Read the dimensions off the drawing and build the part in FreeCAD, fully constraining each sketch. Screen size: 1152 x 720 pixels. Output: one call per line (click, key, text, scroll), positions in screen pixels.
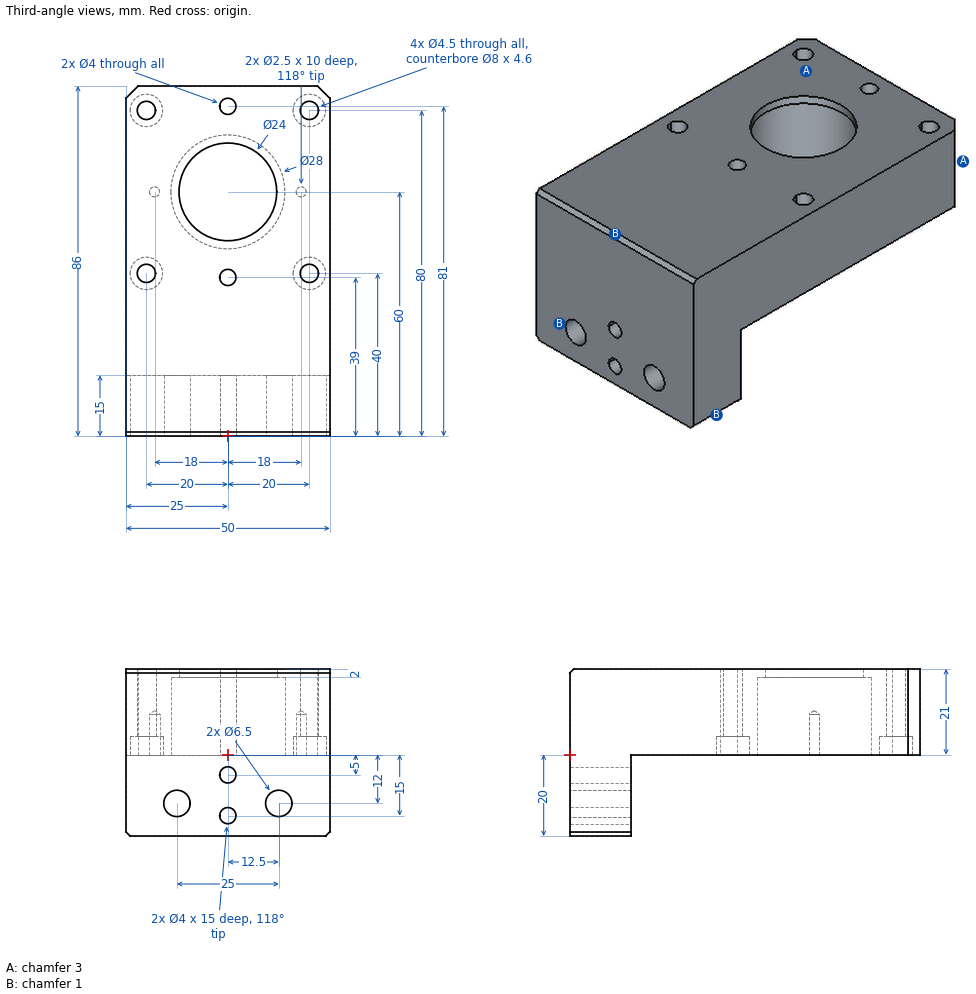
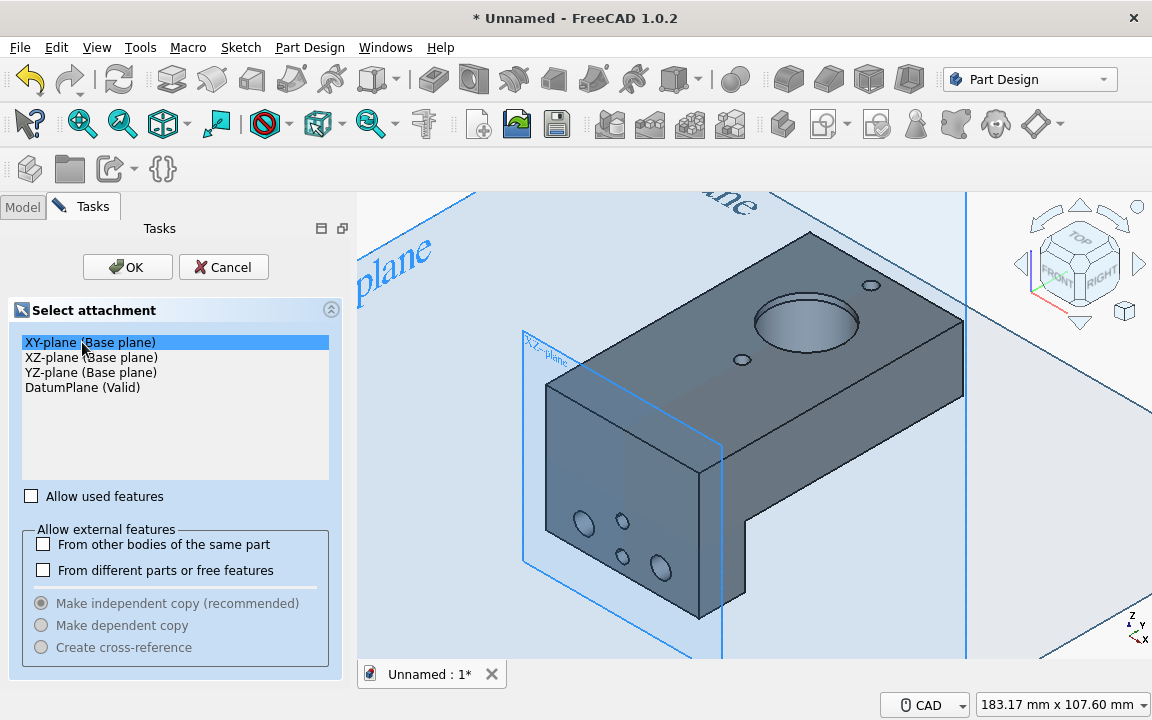
click(128, 267)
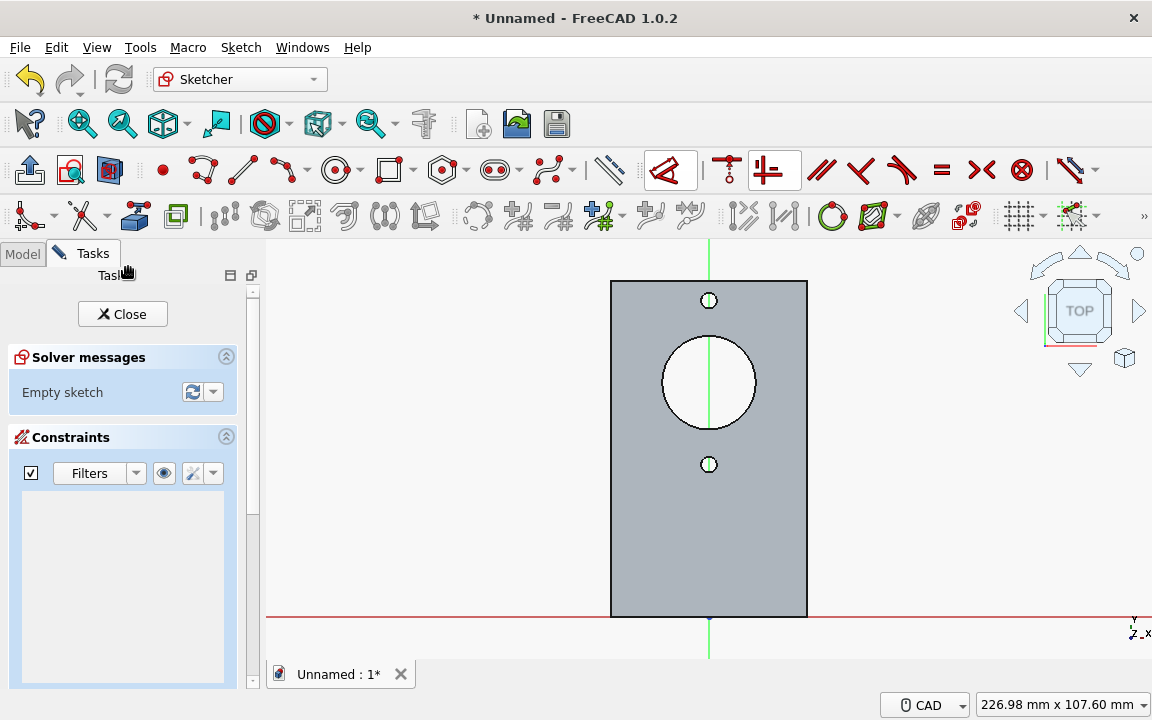
click(110, 170)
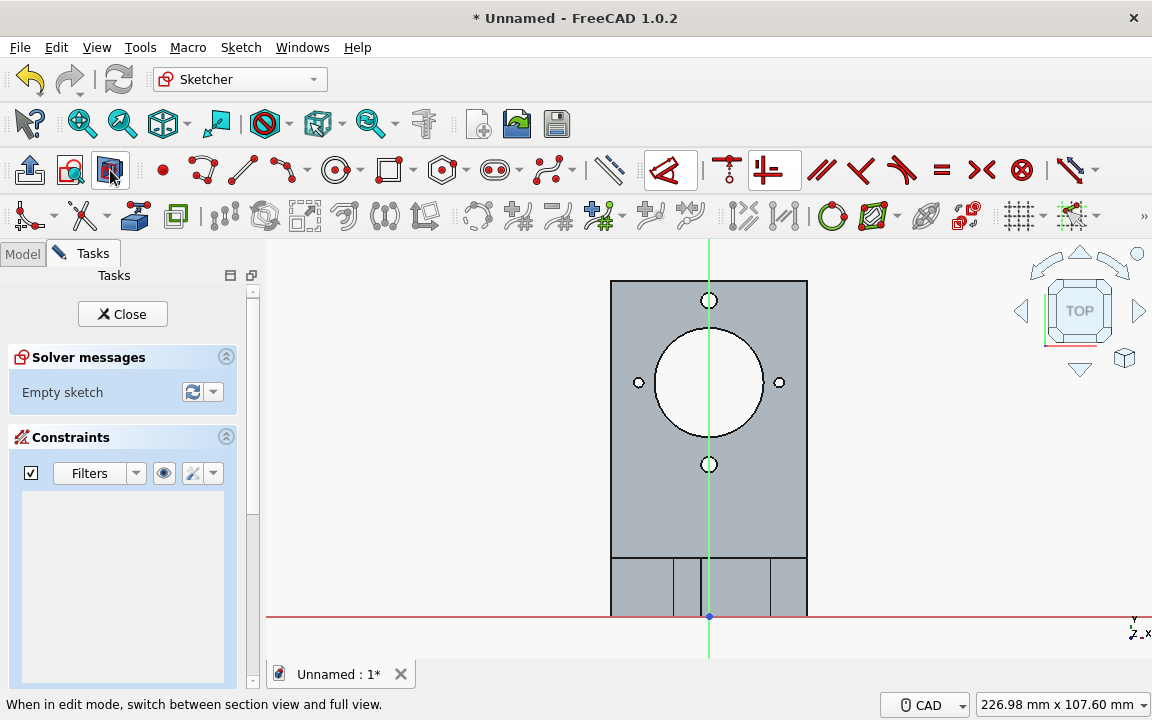
scroll(331, 416, down, 1)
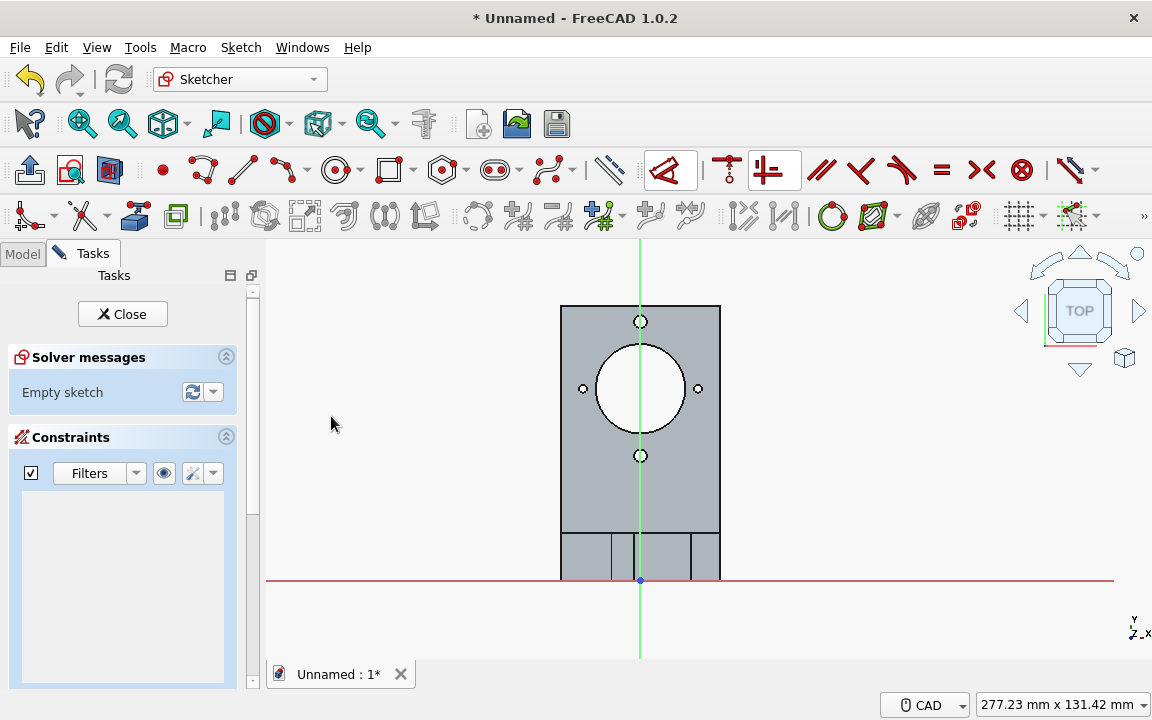
click(336, 170)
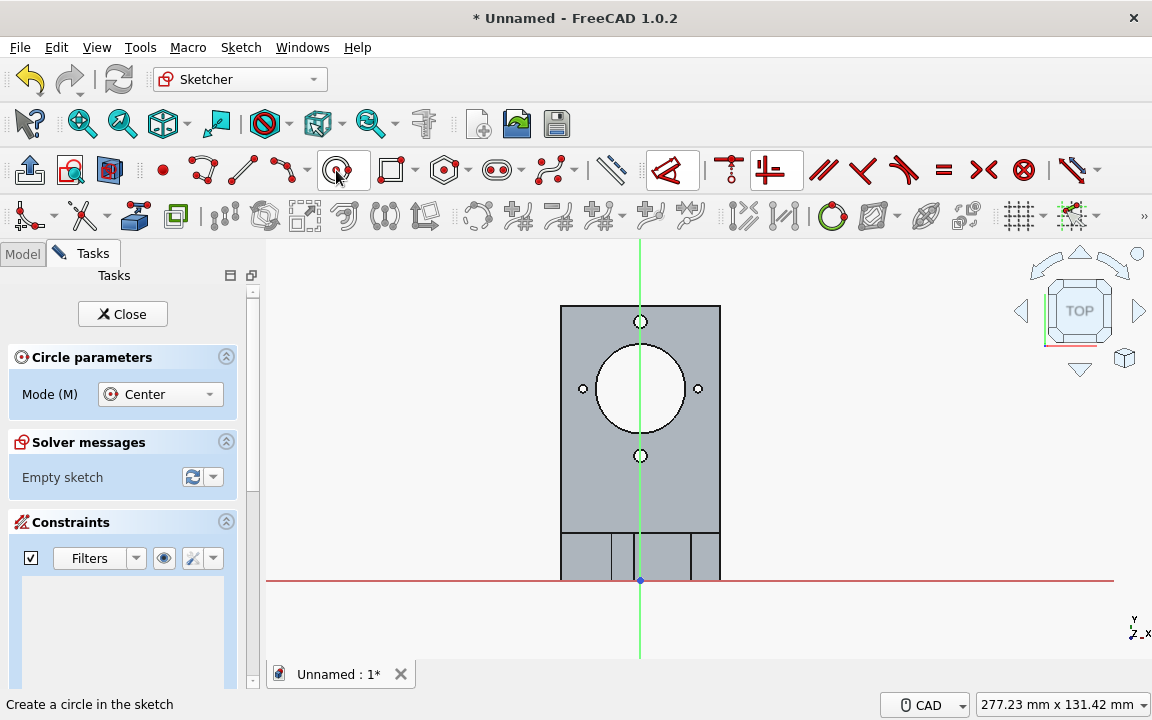
scroll(704, 325, up, 6)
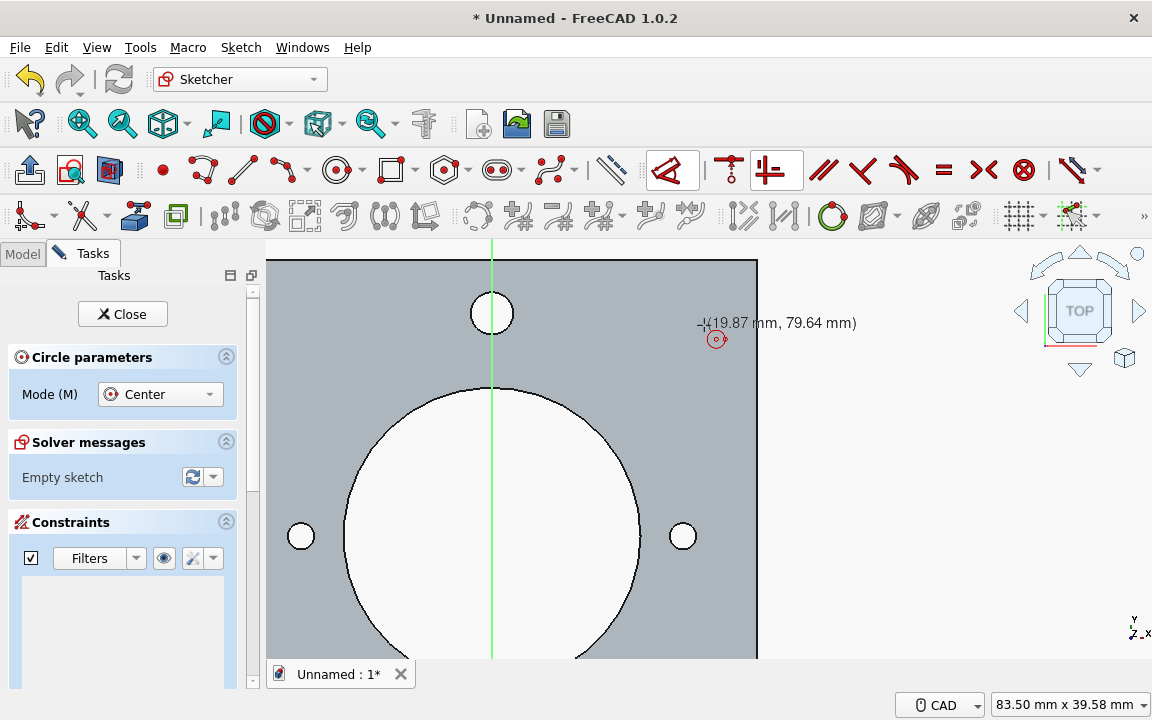
click(704, 324)
click(721, 307)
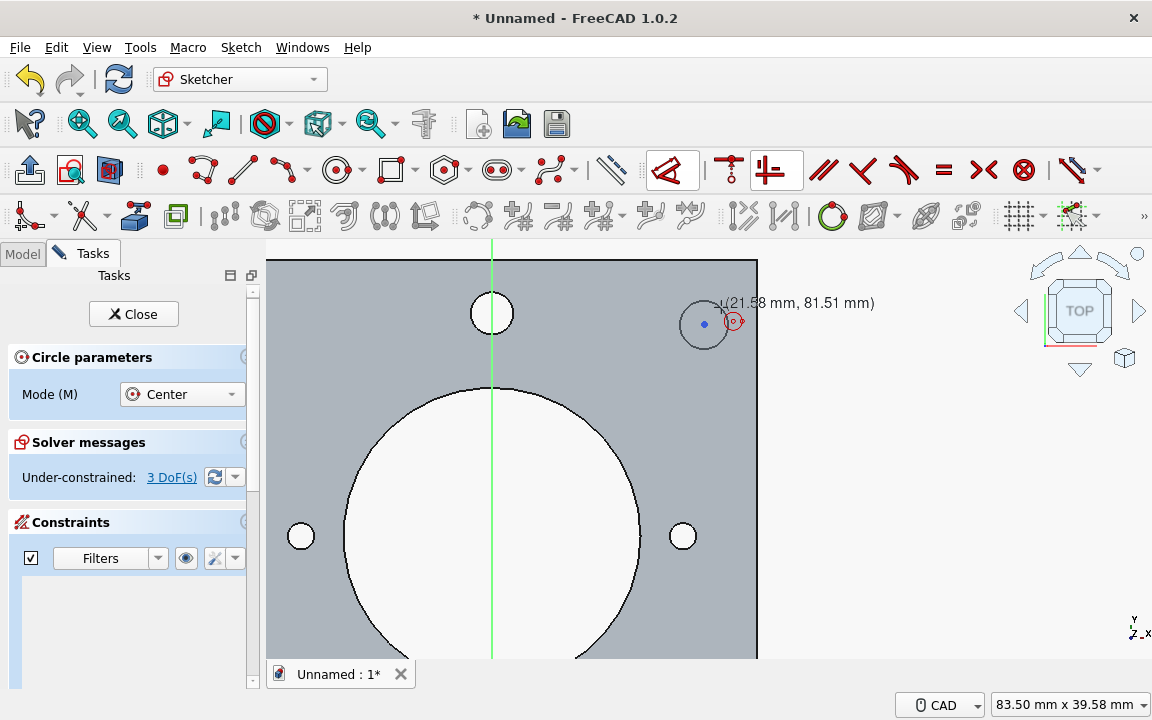
scroll(705, 325, down, 6)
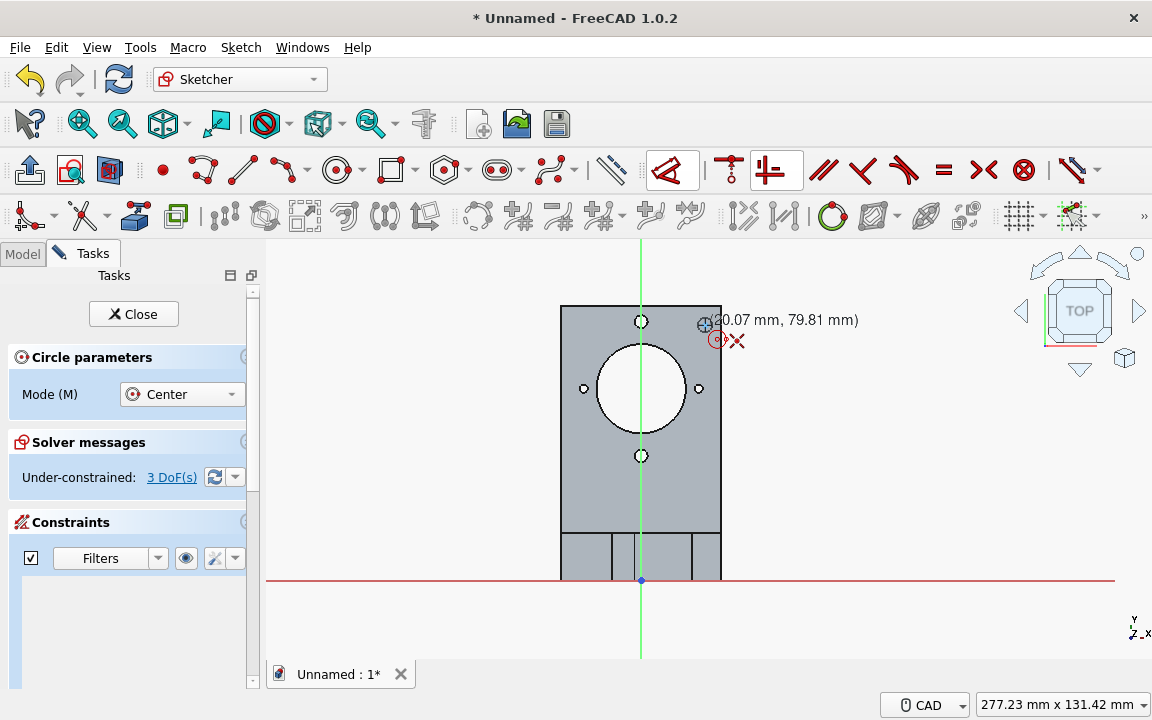
scroll(705, 453, up, 6)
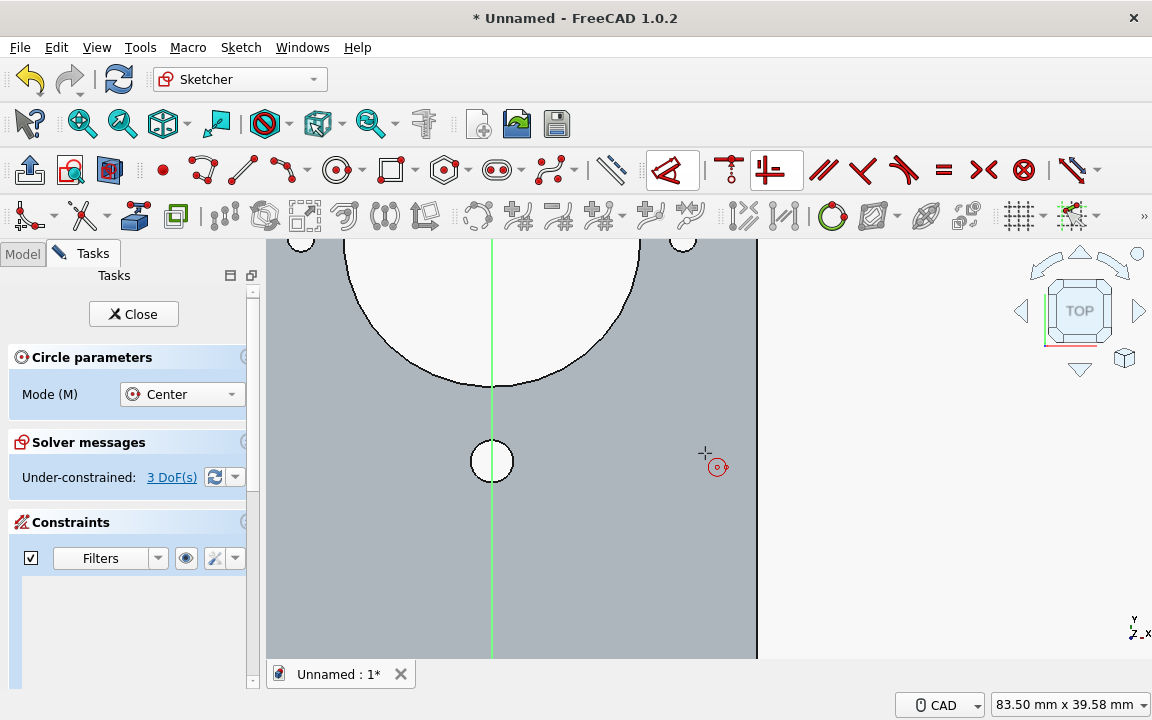
click(704, 451)
click(721, 434)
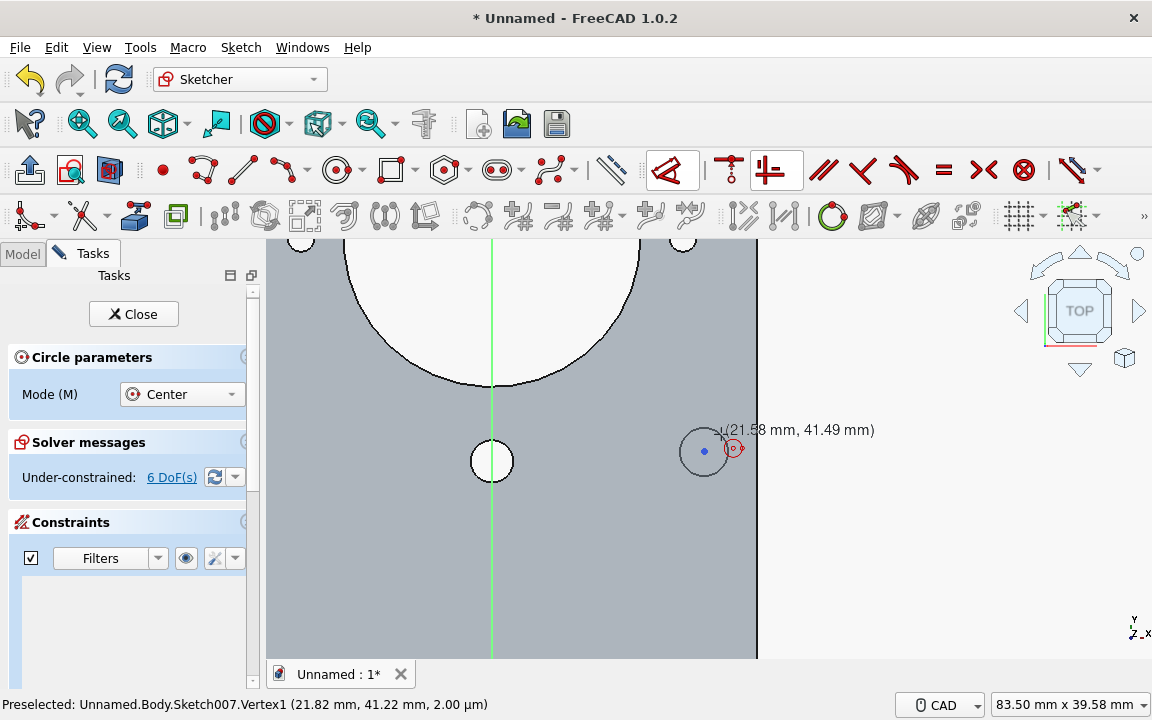
scroll(705, 453, down, 6)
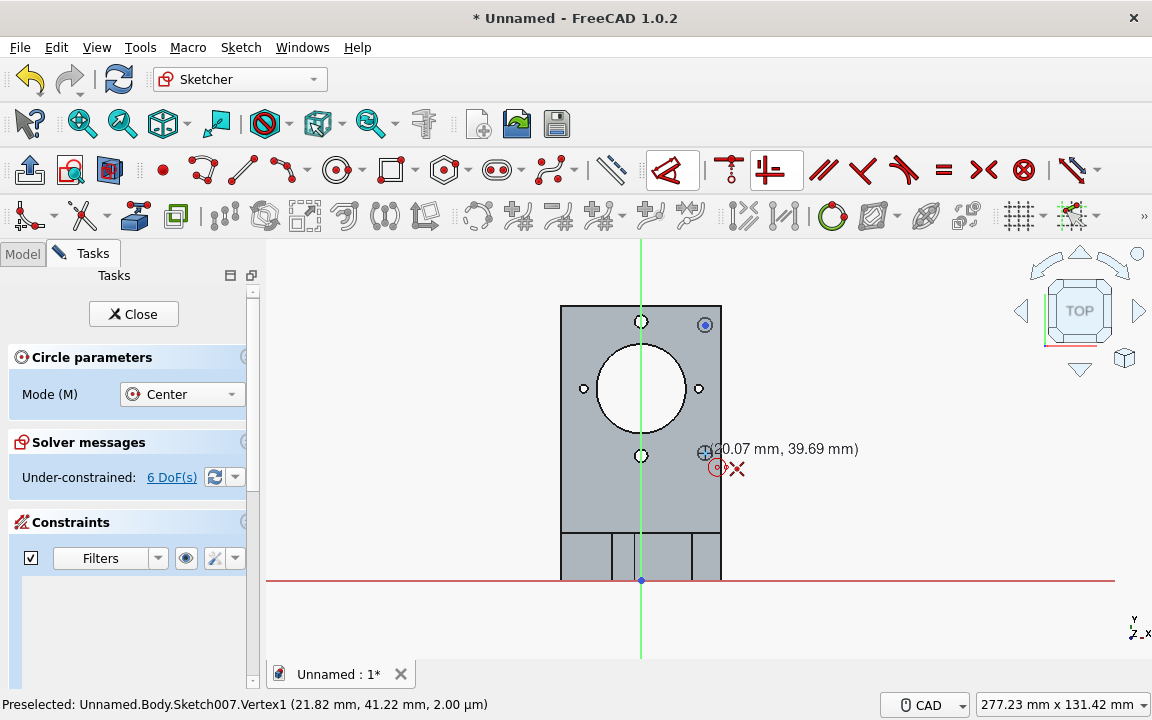
scroll(577, 453, up, 6)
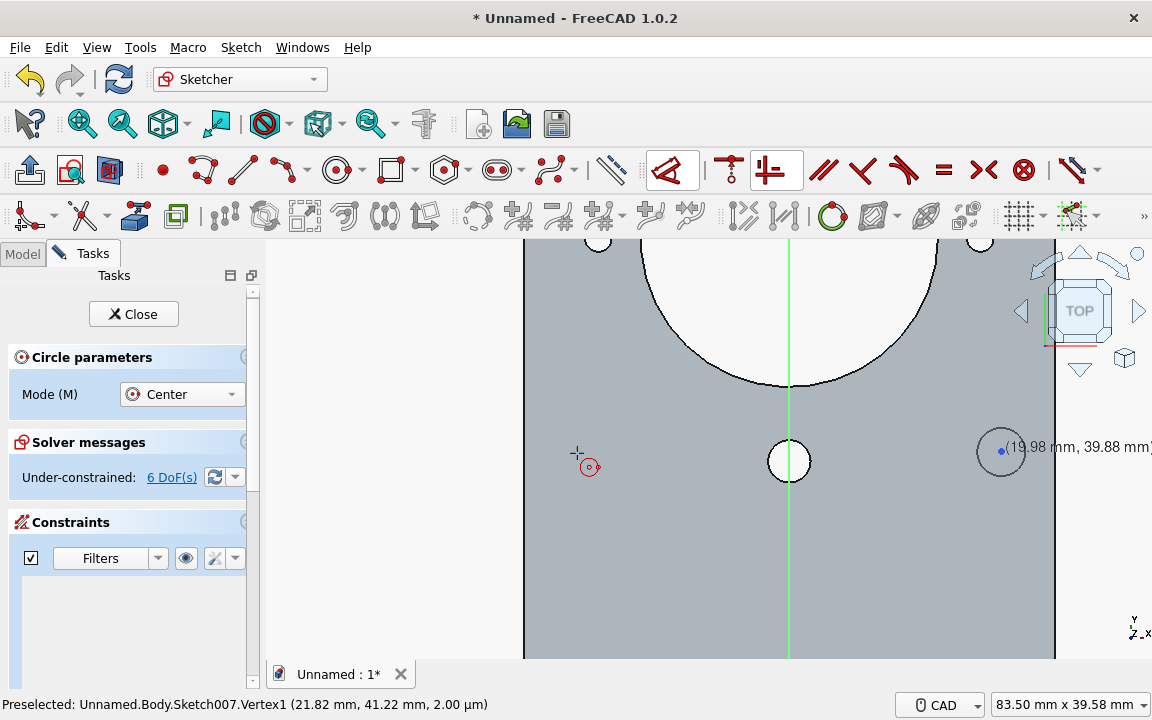
click(577, 451)
click(594, 434)